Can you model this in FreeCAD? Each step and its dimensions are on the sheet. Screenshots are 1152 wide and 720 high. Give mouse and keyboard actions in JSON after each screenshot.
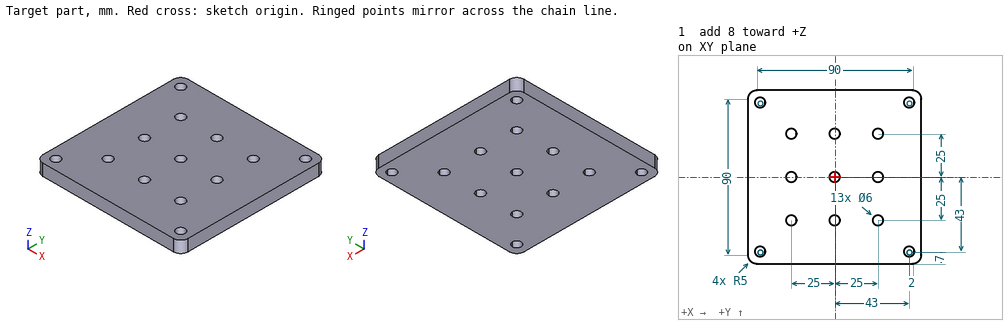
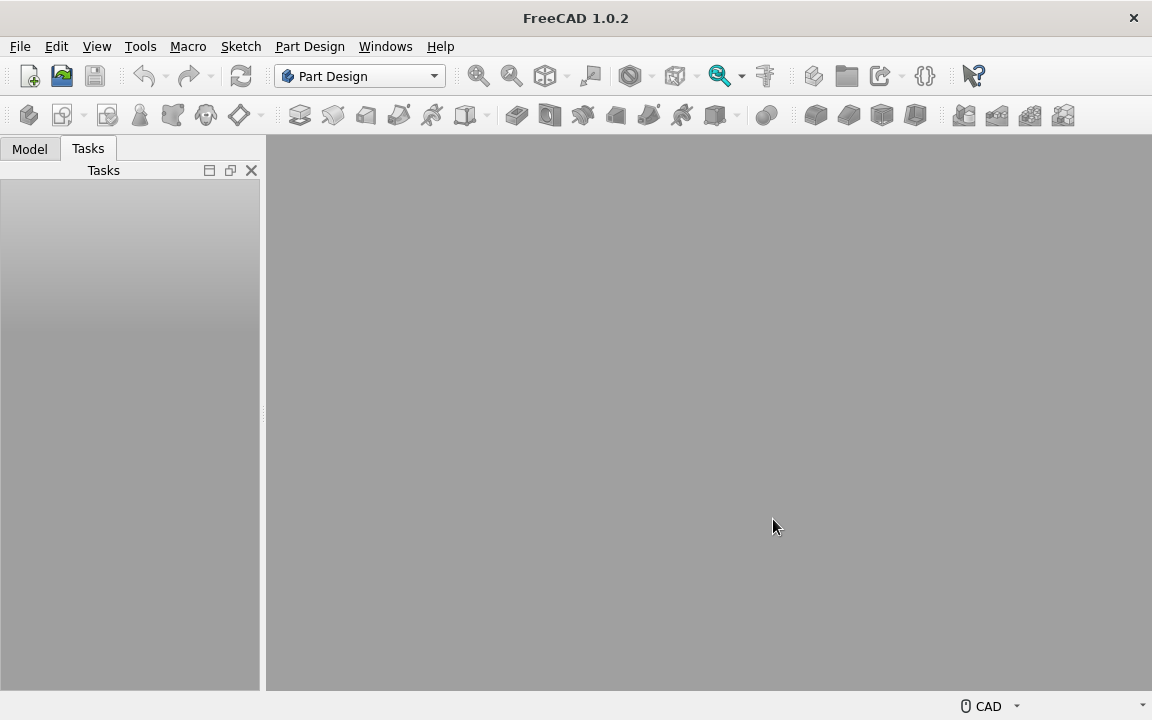
{"action": "left_click", "coordinate": [29, 76]}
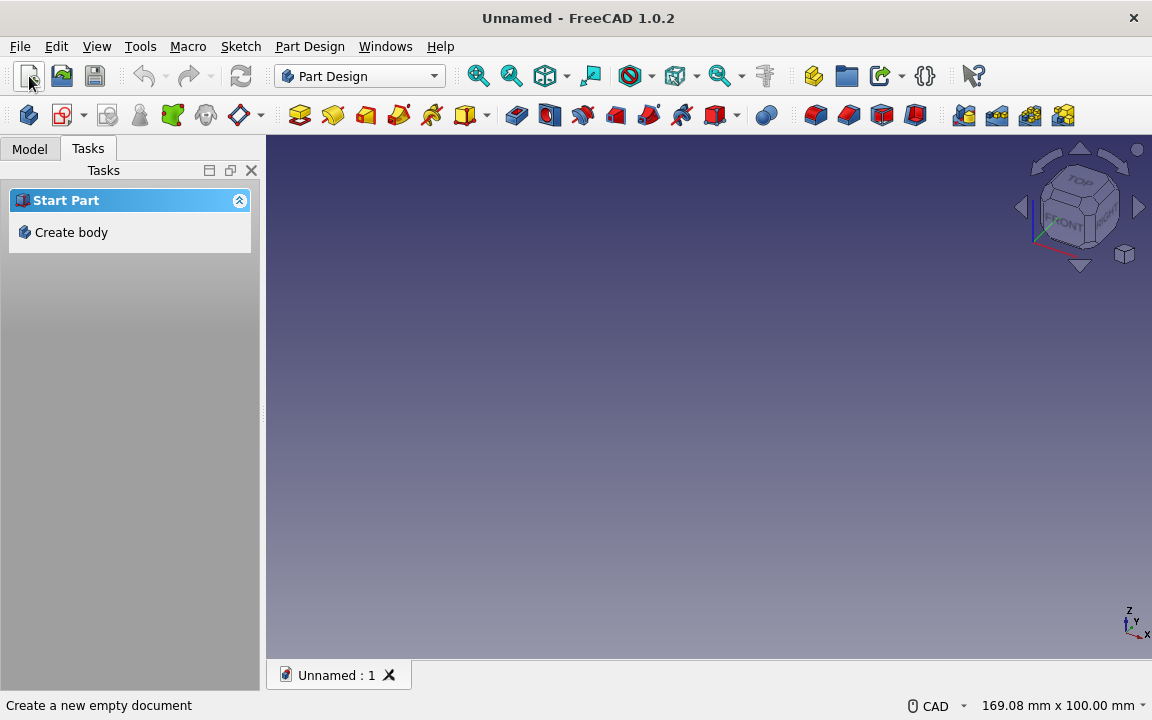
{"action": "left_click", "coordinate": [62, 116]}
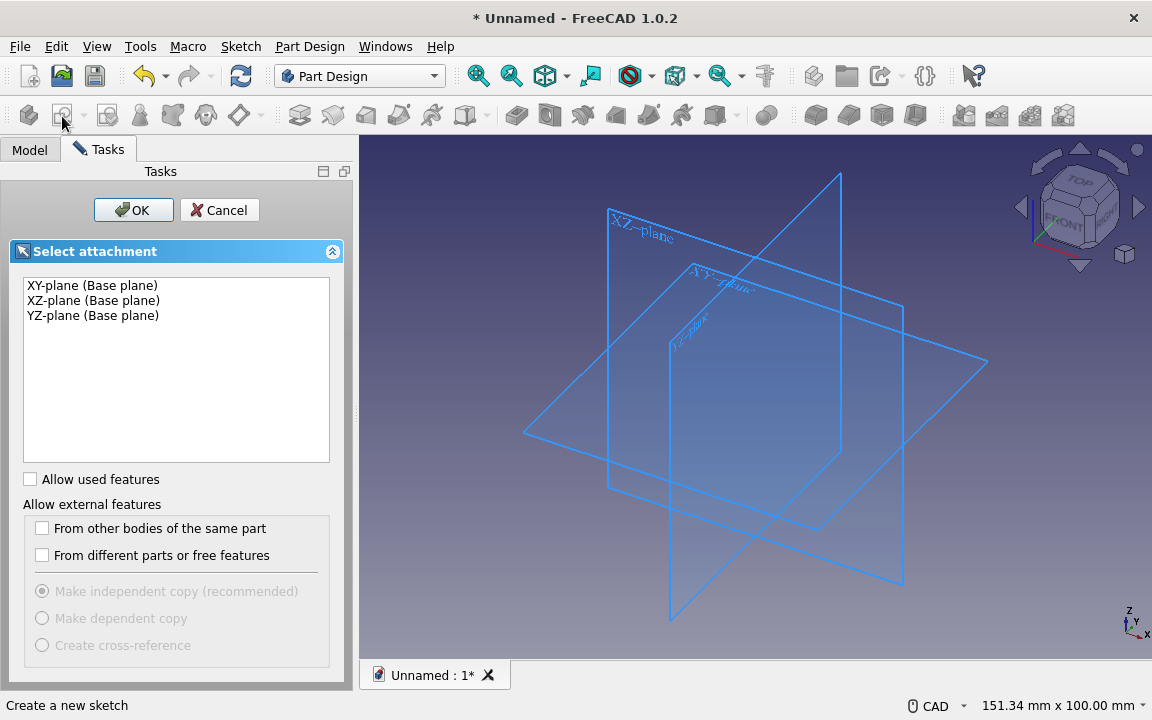
{"action": "left_click", "coordinate": [84, 286]}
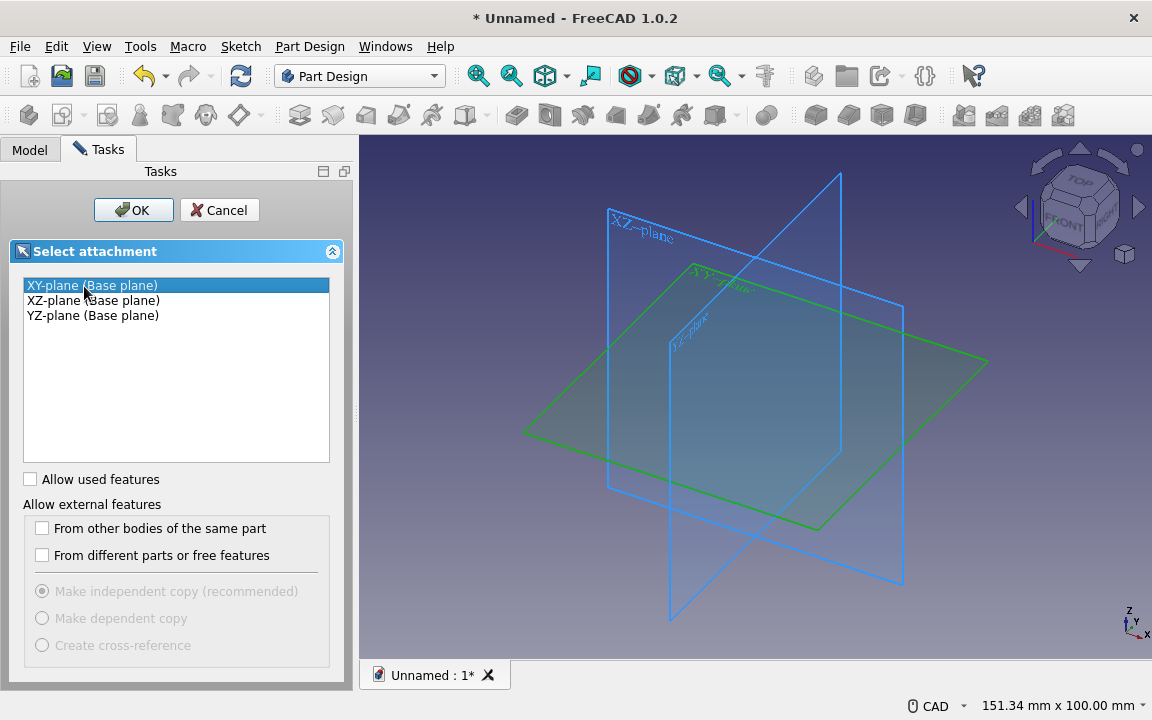
{"action": "left_click", "coordinate": [134, 210]}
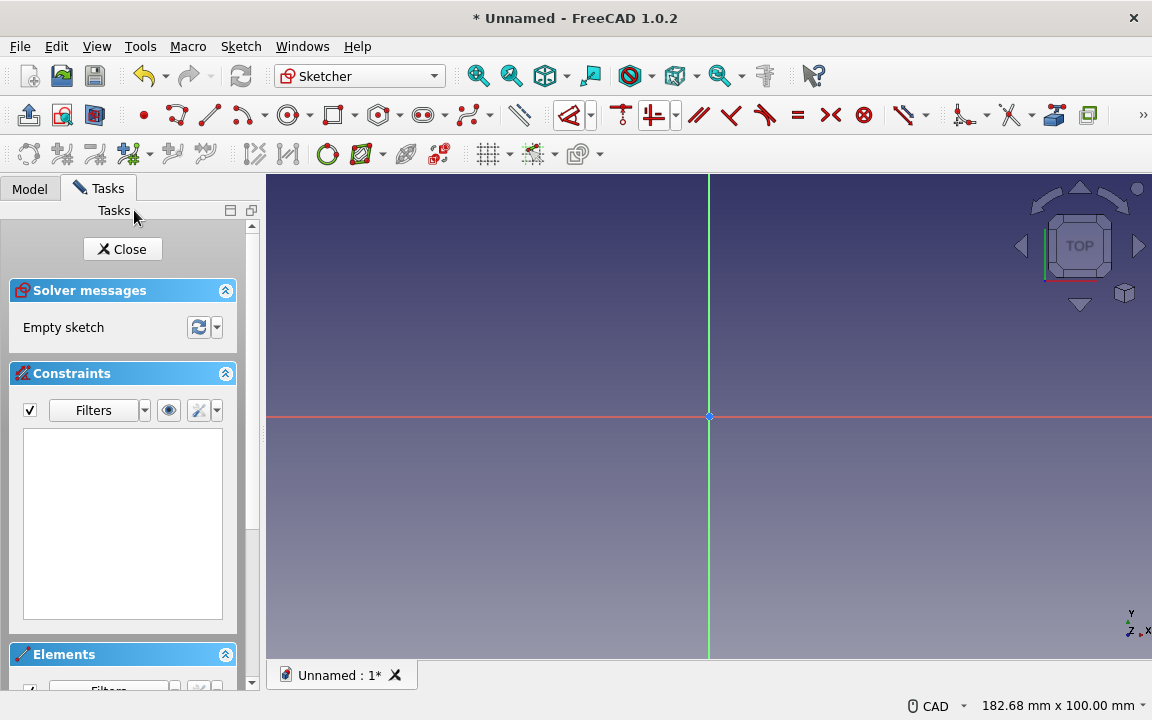
{"action": "scroll", "coordinate": [501, 416], "scroll_direction": "down", "scroll_amount": 2}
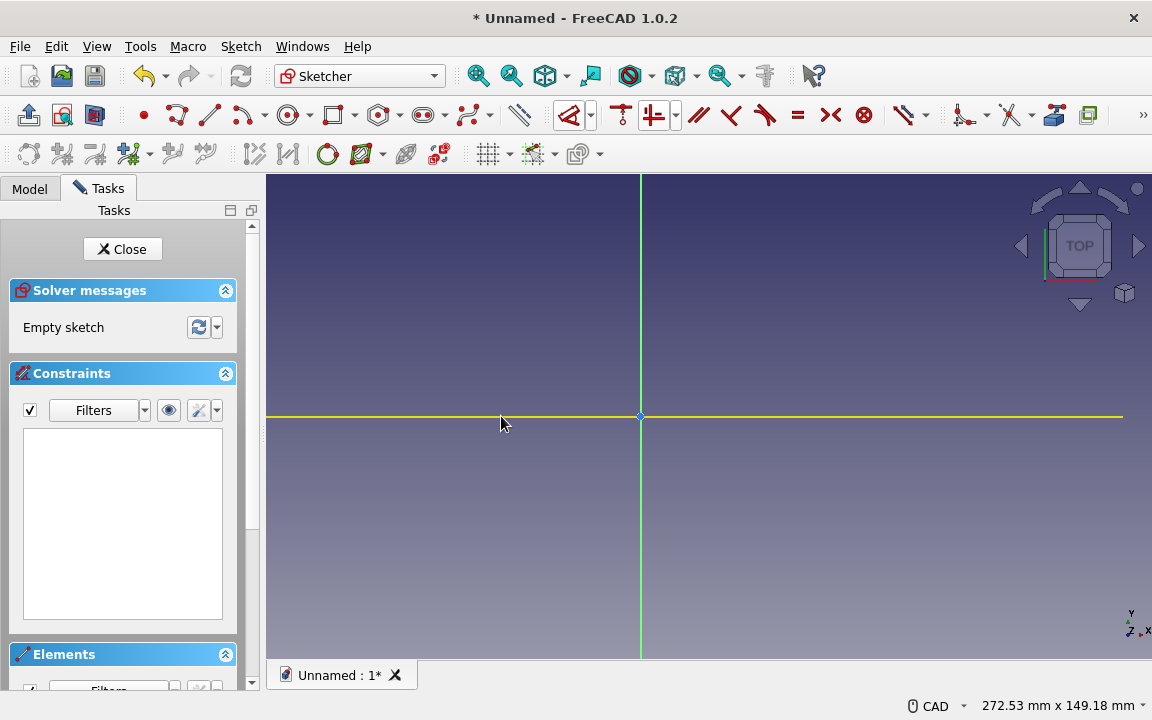
{"action": "left_click", "coordinate": [210, 116]}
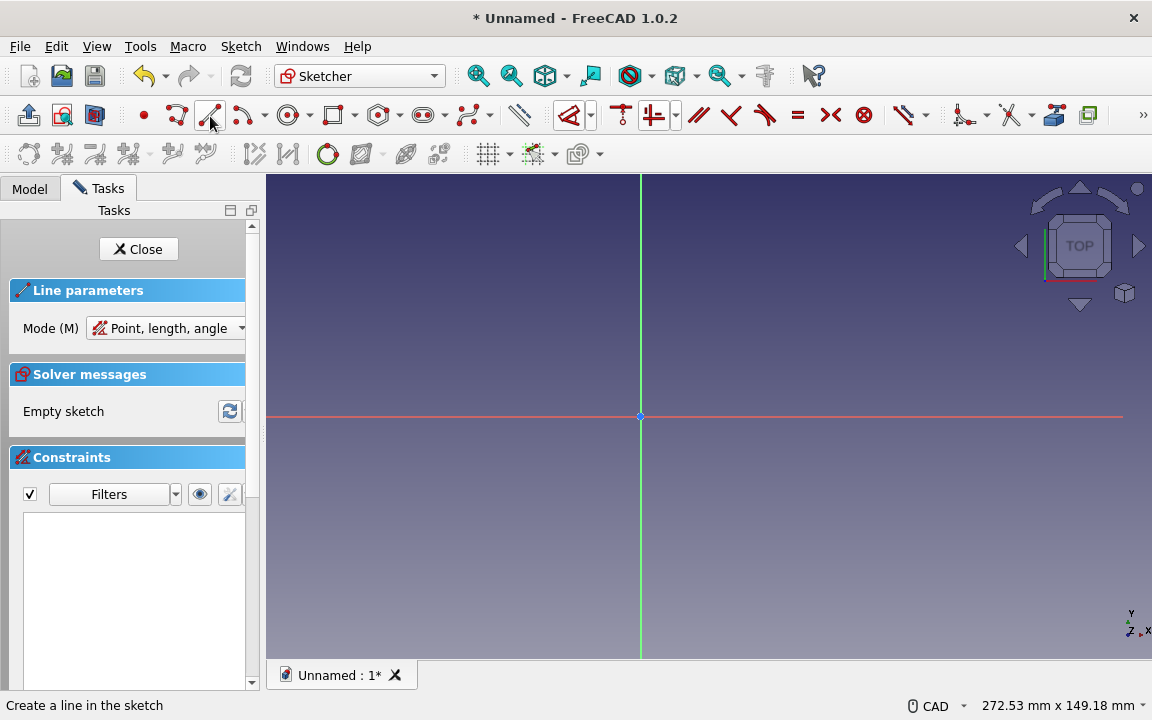
{"action": "left_click", "coordinate": [787, 254]}
{"action": "left_click", "coordinate": [494, 254]}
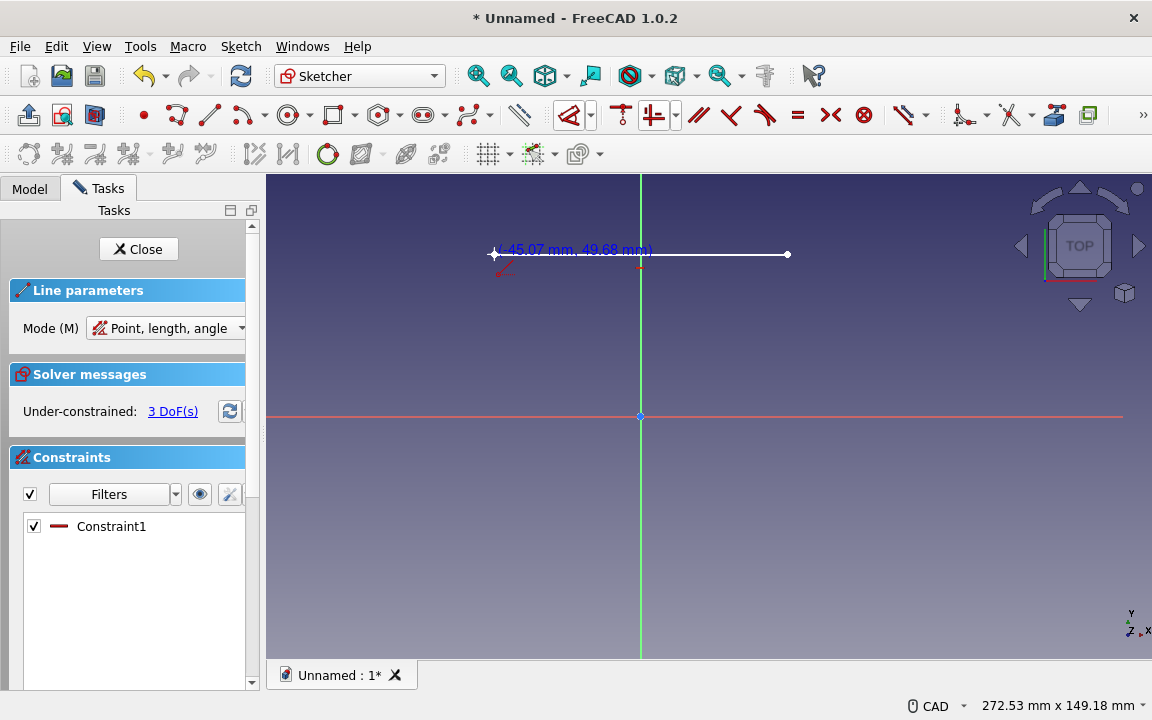
{"action": "left_click", "coordinate": [478, 270]}
{"action": "left_click", "coordinate": [478, 563]}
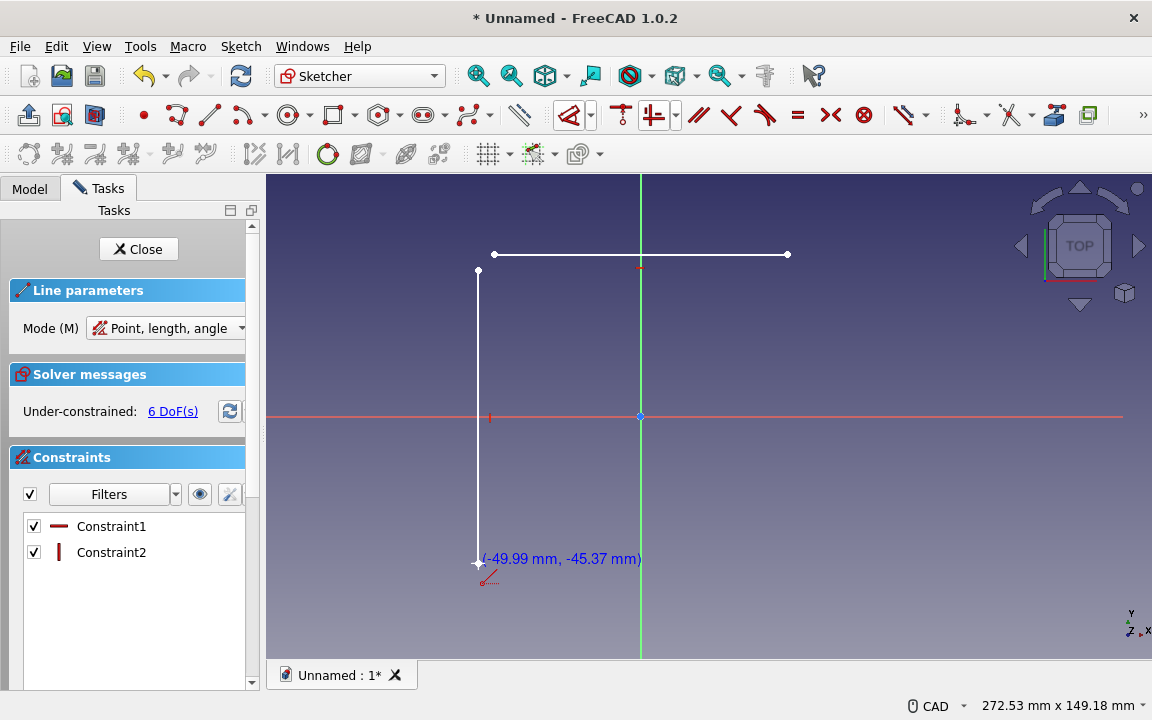
{"action": "left_click", "coordinate": [494, 579]}
{"action": "left_click", "coordinate": [787, 579]}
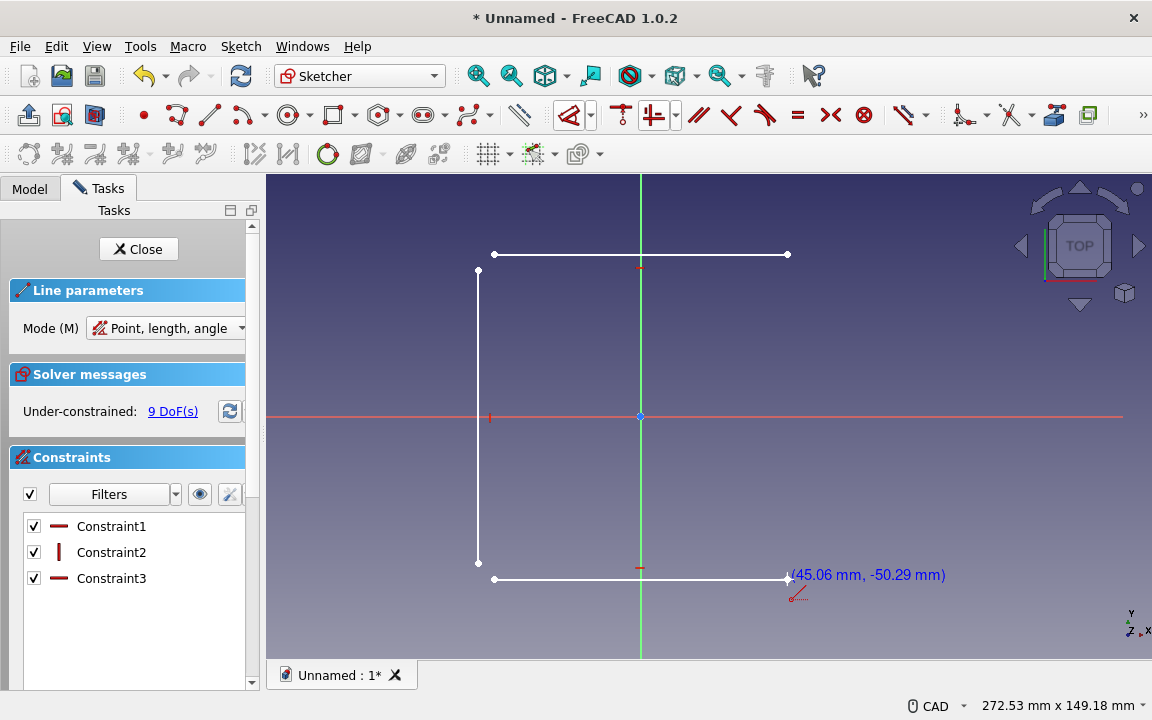
{"action": "left_click", "coordinate": [803, 563]}
{"action": "left_click", "coordinate": [803, 270]}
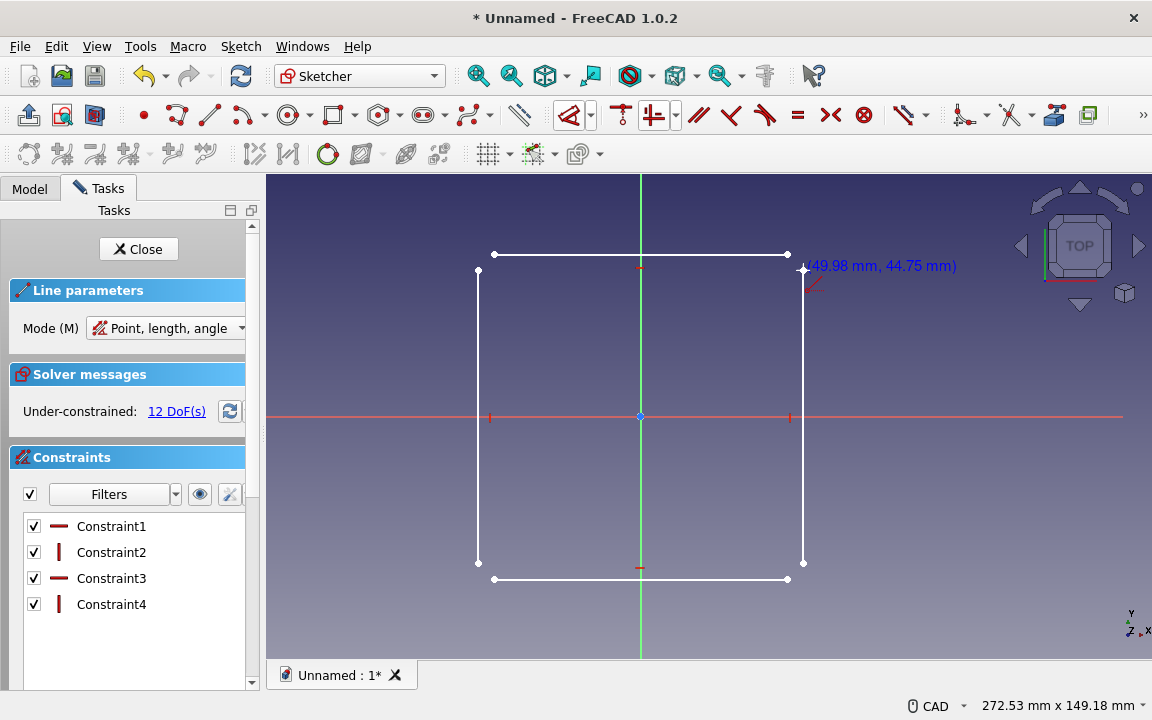
{"action": "key", "text": "g 3 a"}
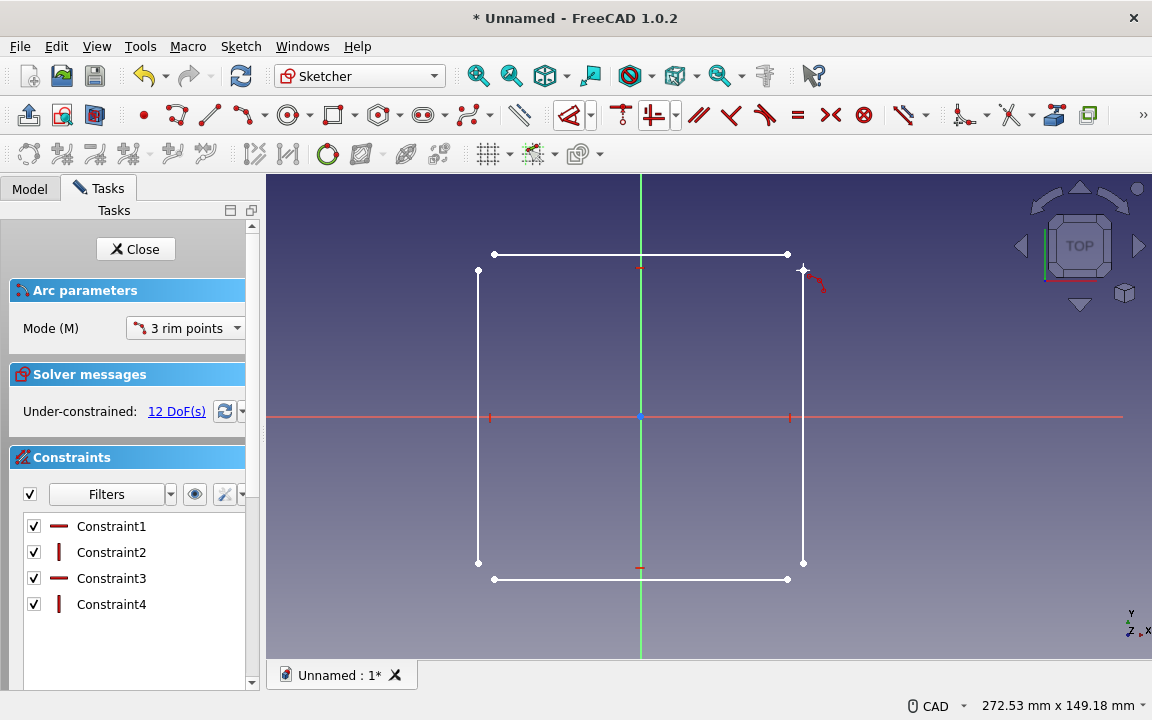
{"action": "left_click", "coordinate": [494, 255]}
{"action": "left_click", "coordinate": [478, 271]}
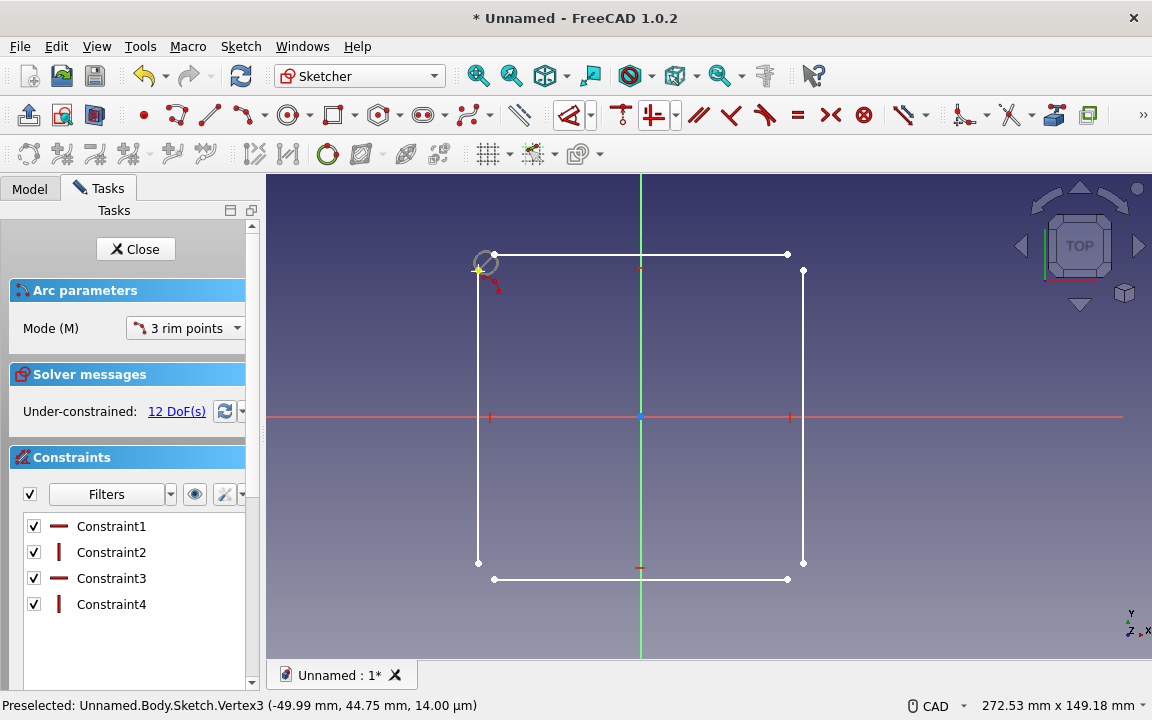
{"action": "scroll", "coordinate": [483, 259], "scroll_direction": "up", "scroll_amount": 7}